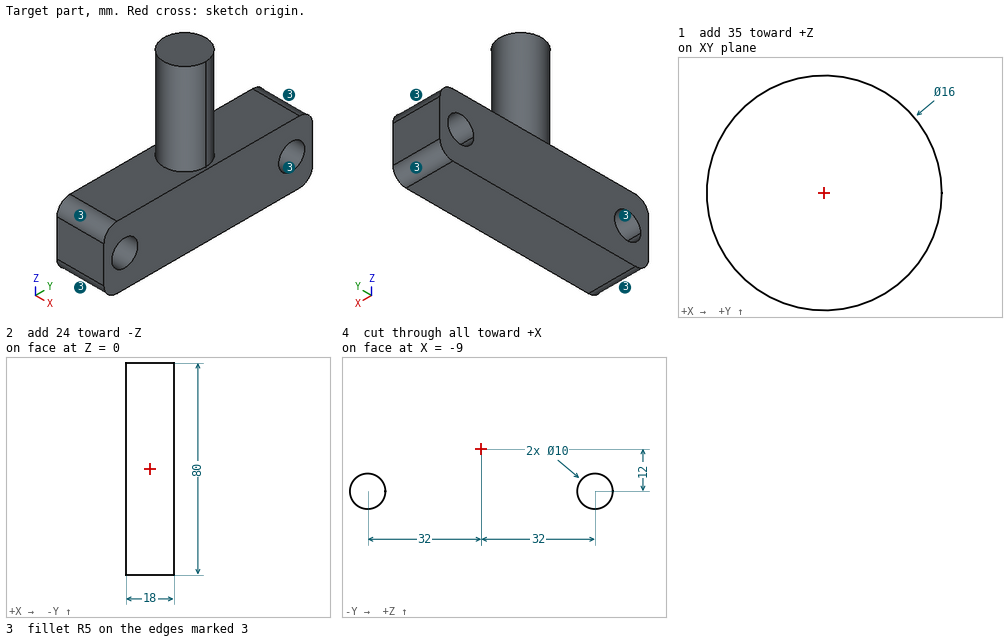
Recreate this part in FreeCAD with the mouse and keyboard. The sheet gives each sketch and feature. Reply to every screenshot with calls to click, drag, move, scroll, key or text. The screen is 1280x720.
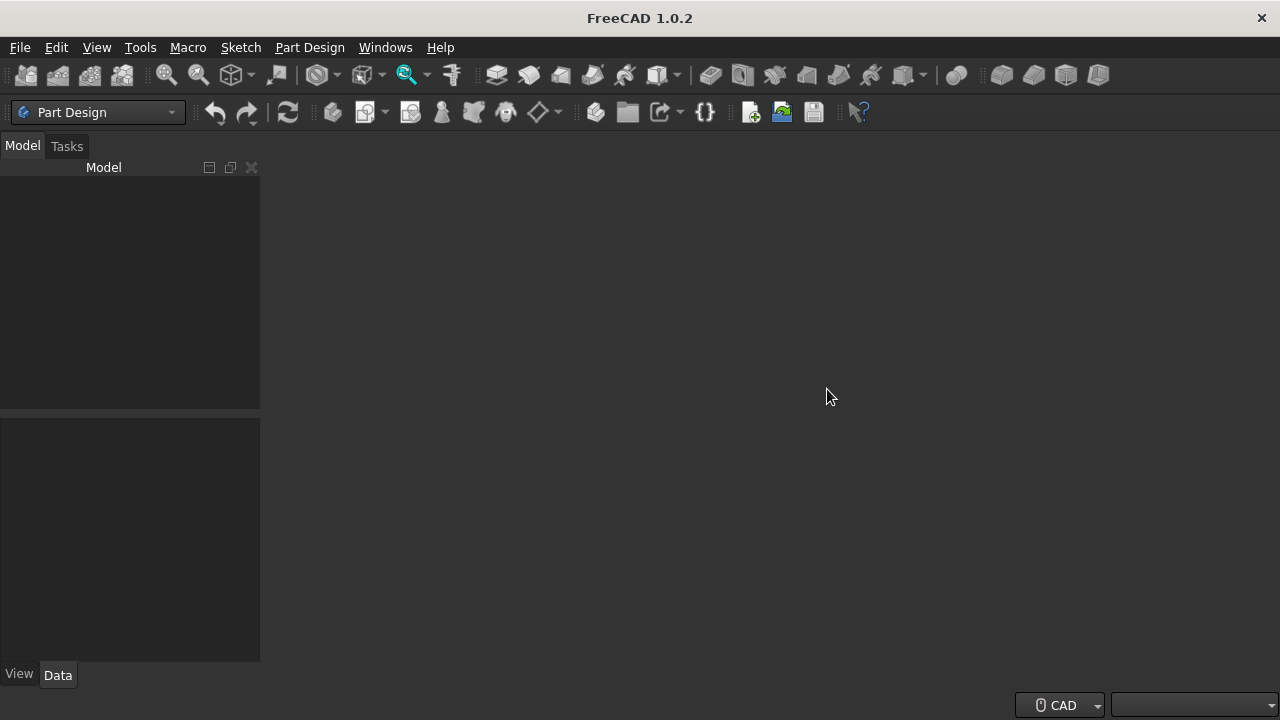
click(750, 112)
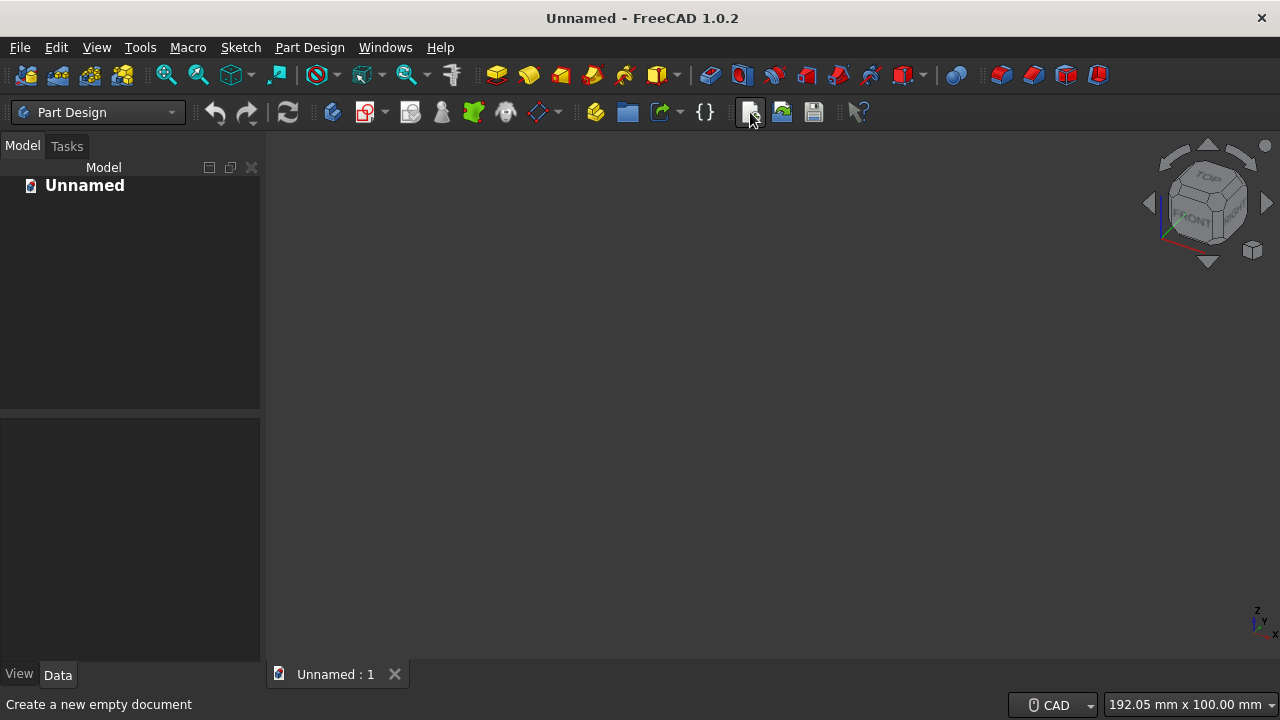
click(366, 112)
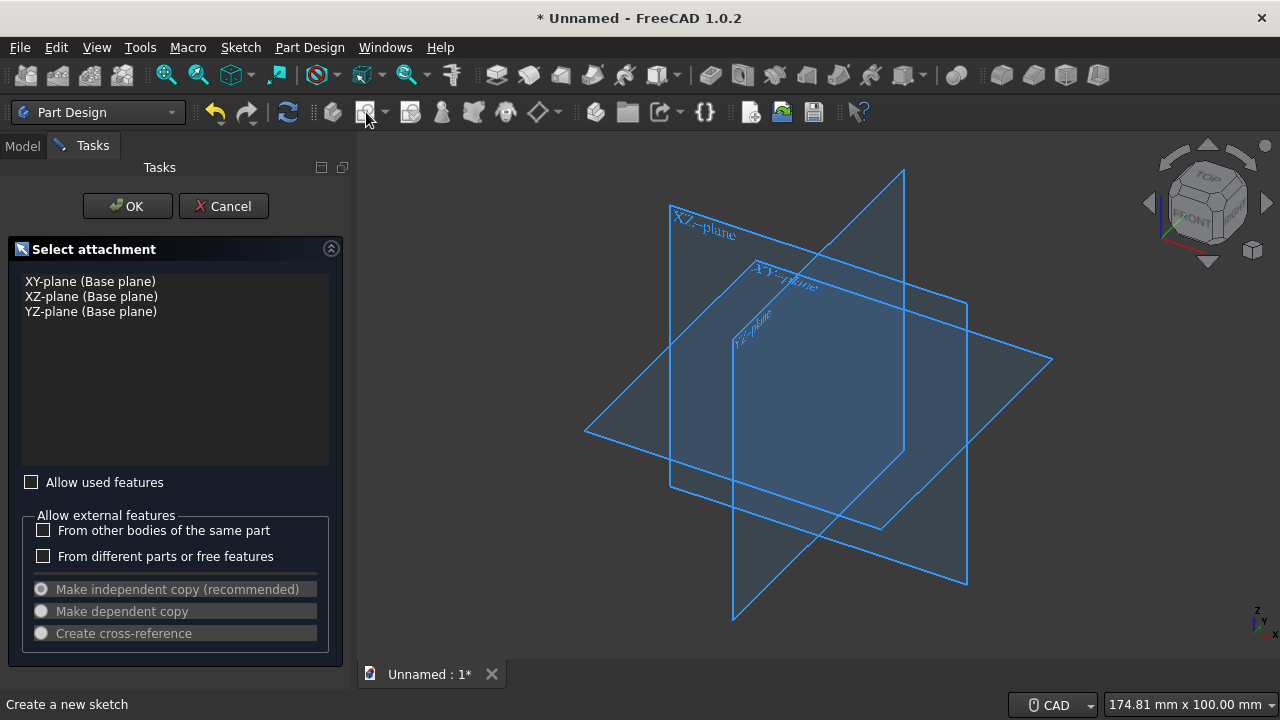
click(82, 282)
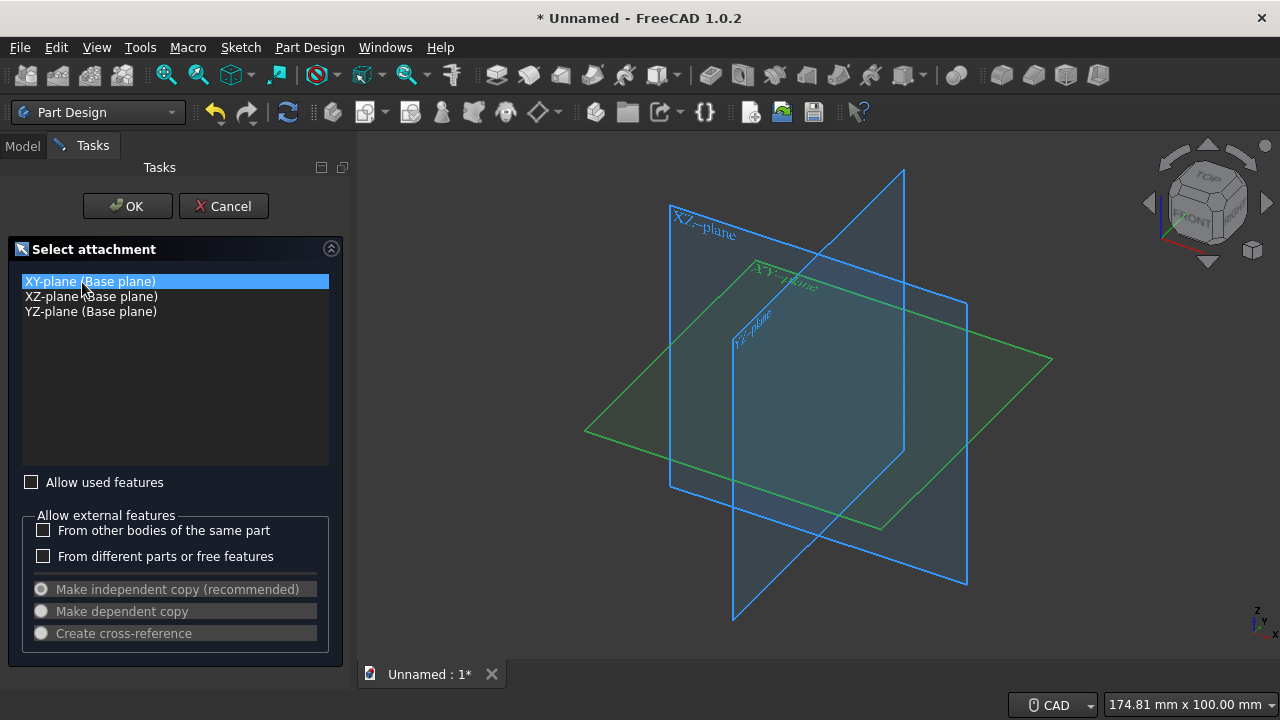
click(128, 206)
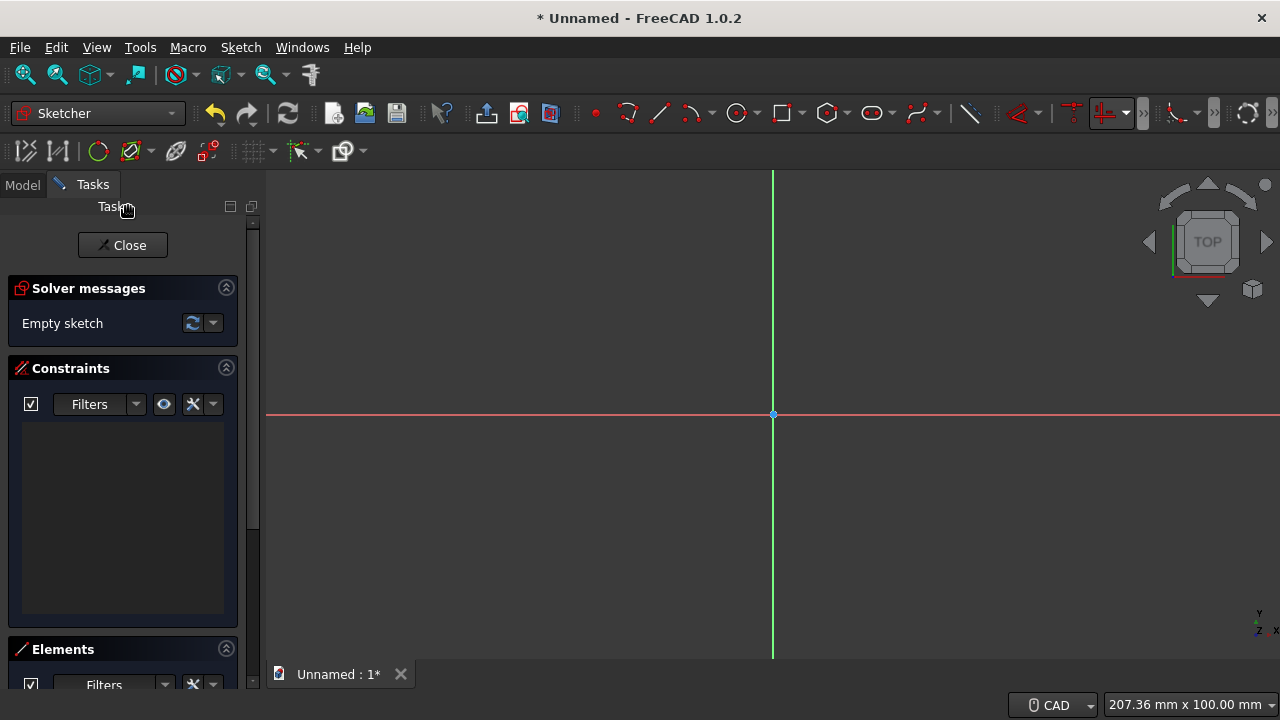
scroll(795, 415, up, 7)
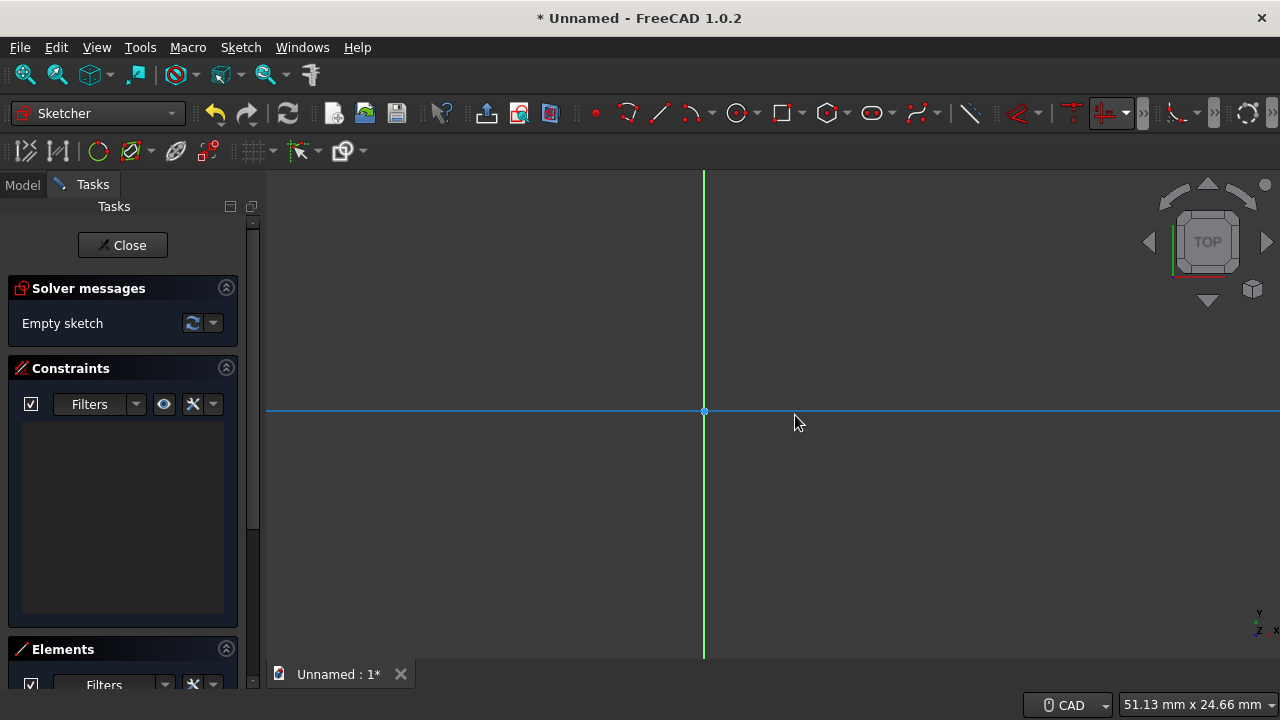
click(738, 114)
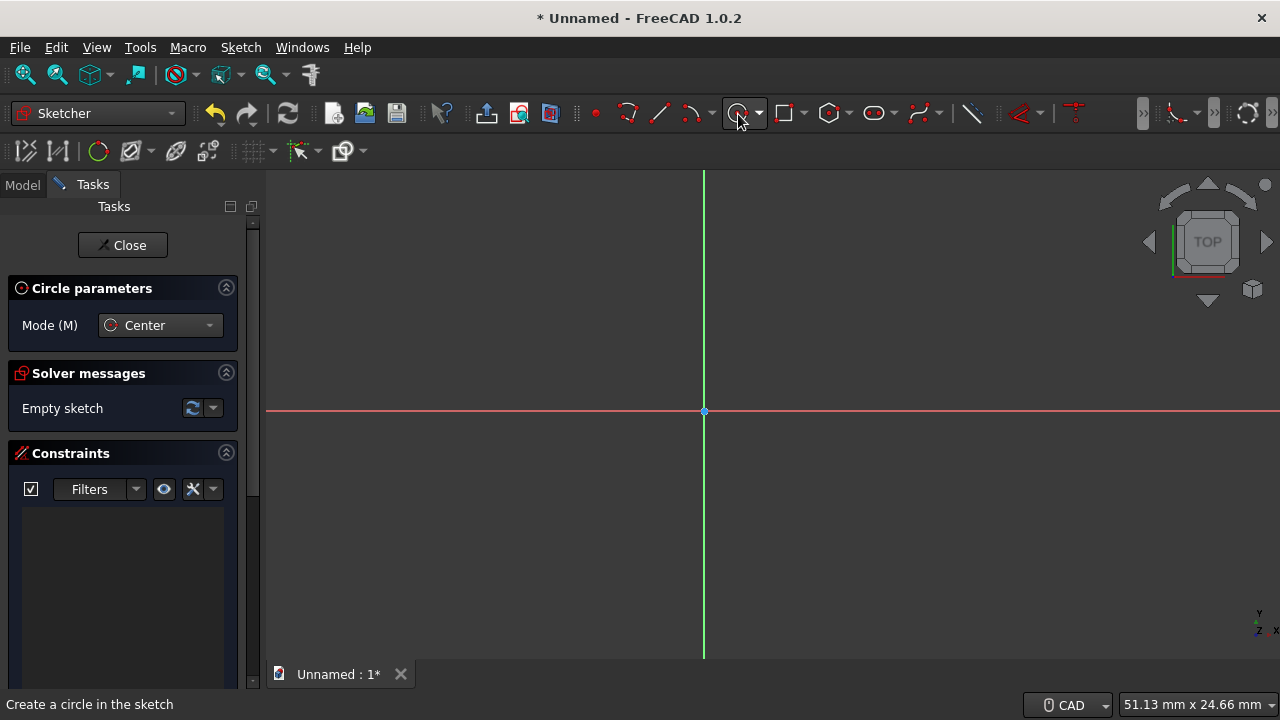
click(704, 411)
move(816, 299)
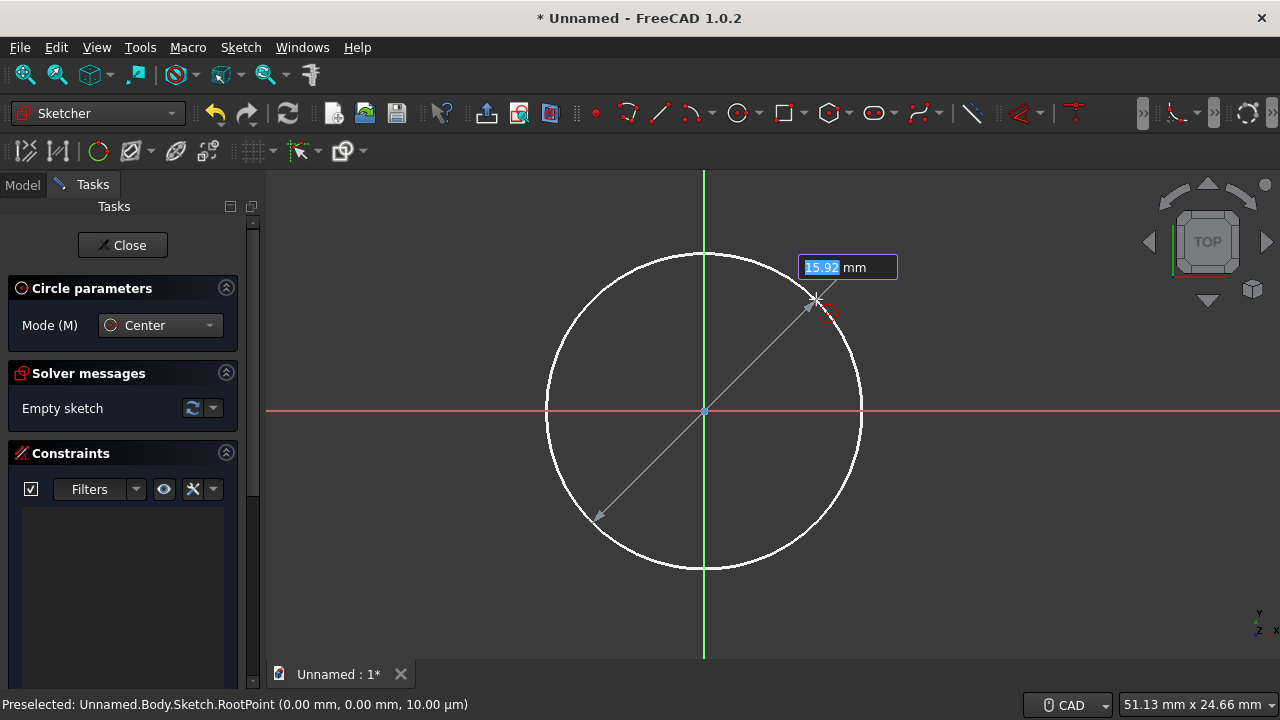
text(16)
key(Return)
key(Escape)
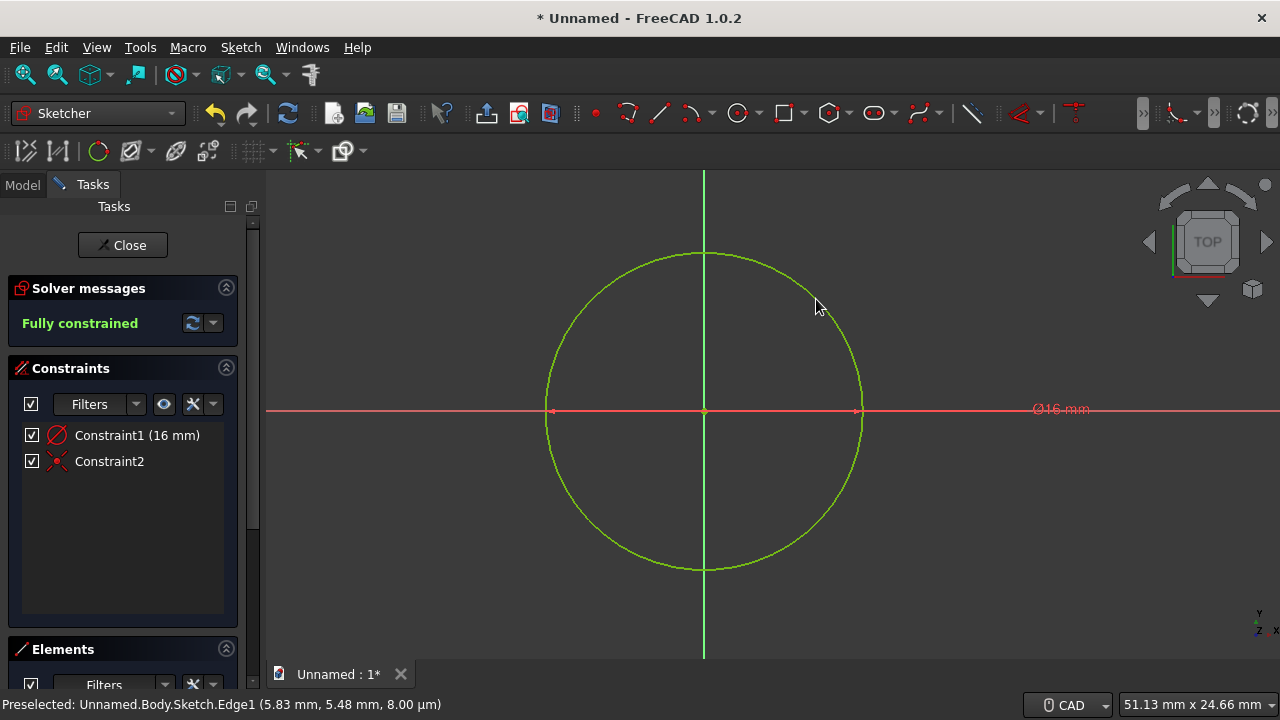
click(123, 245)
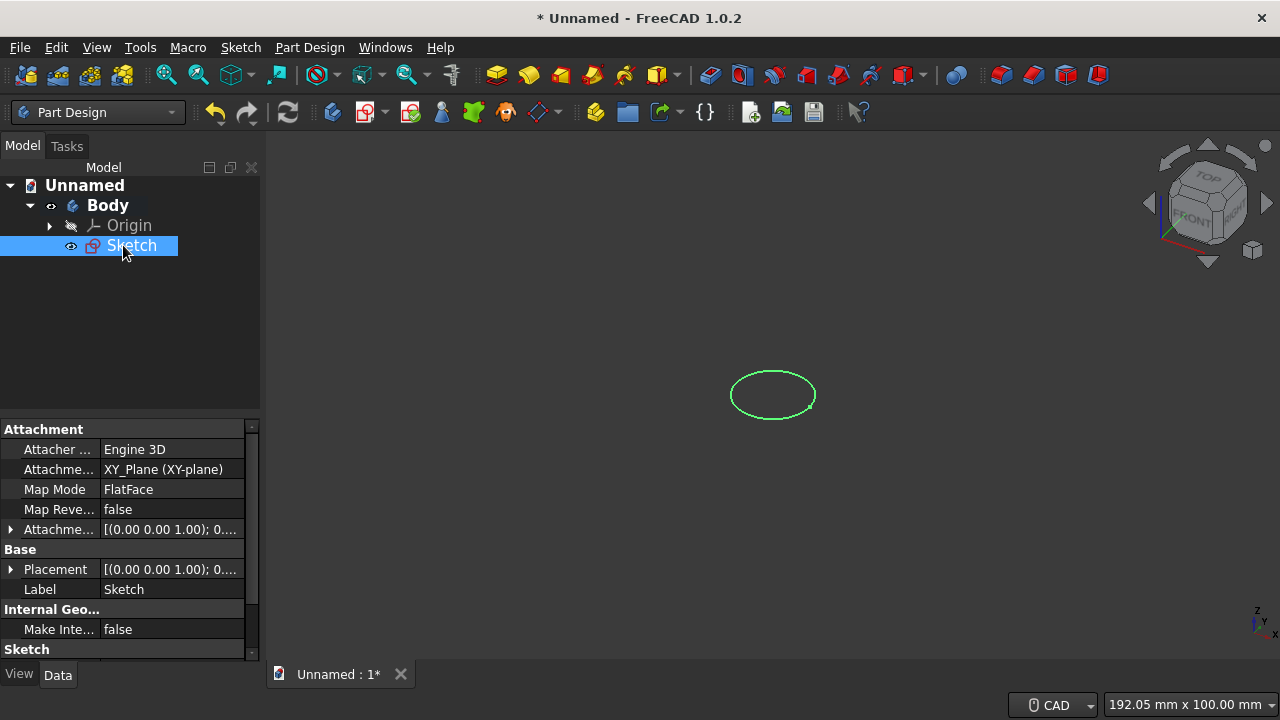
click(498, 76)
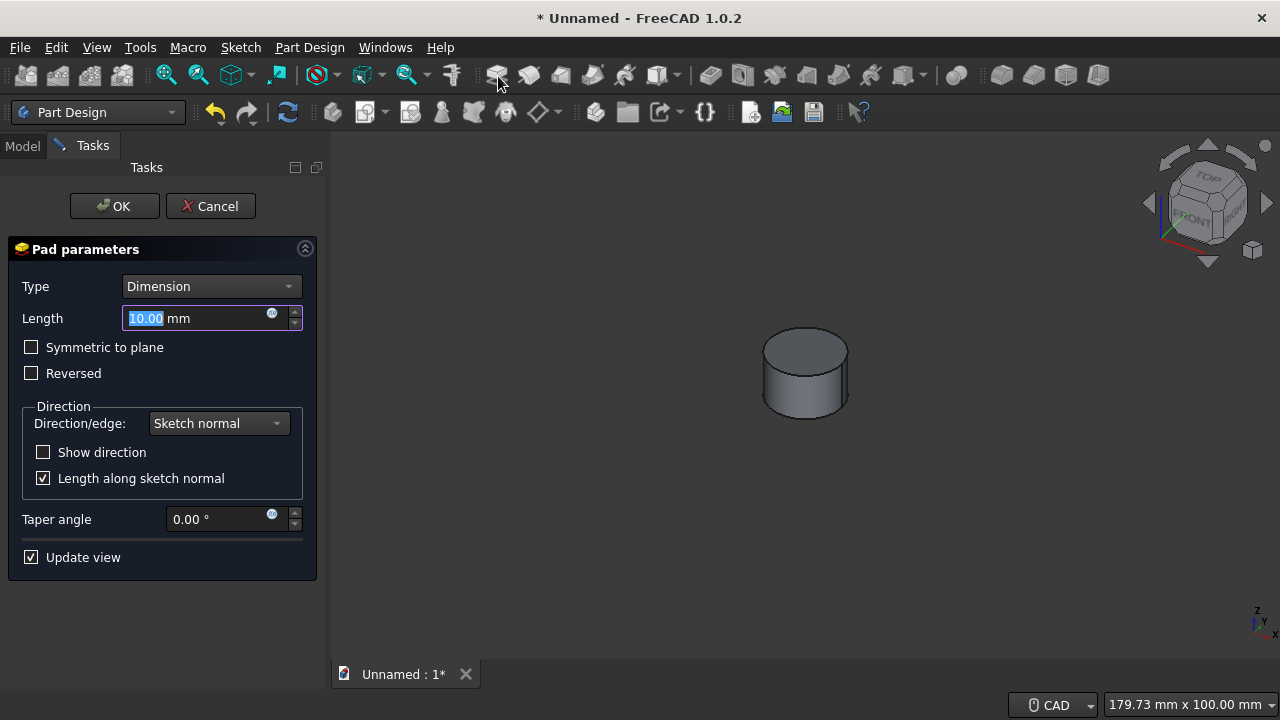
text(35)
key(Tab)